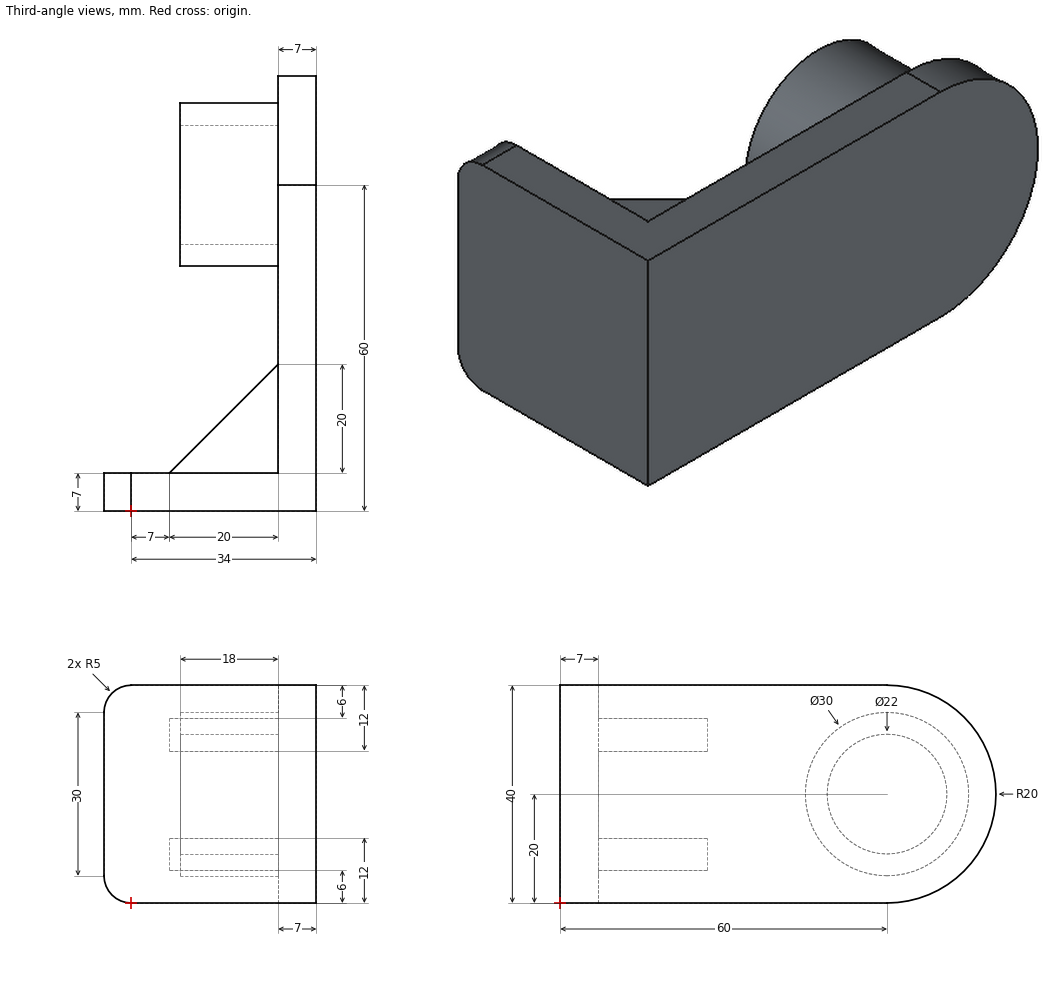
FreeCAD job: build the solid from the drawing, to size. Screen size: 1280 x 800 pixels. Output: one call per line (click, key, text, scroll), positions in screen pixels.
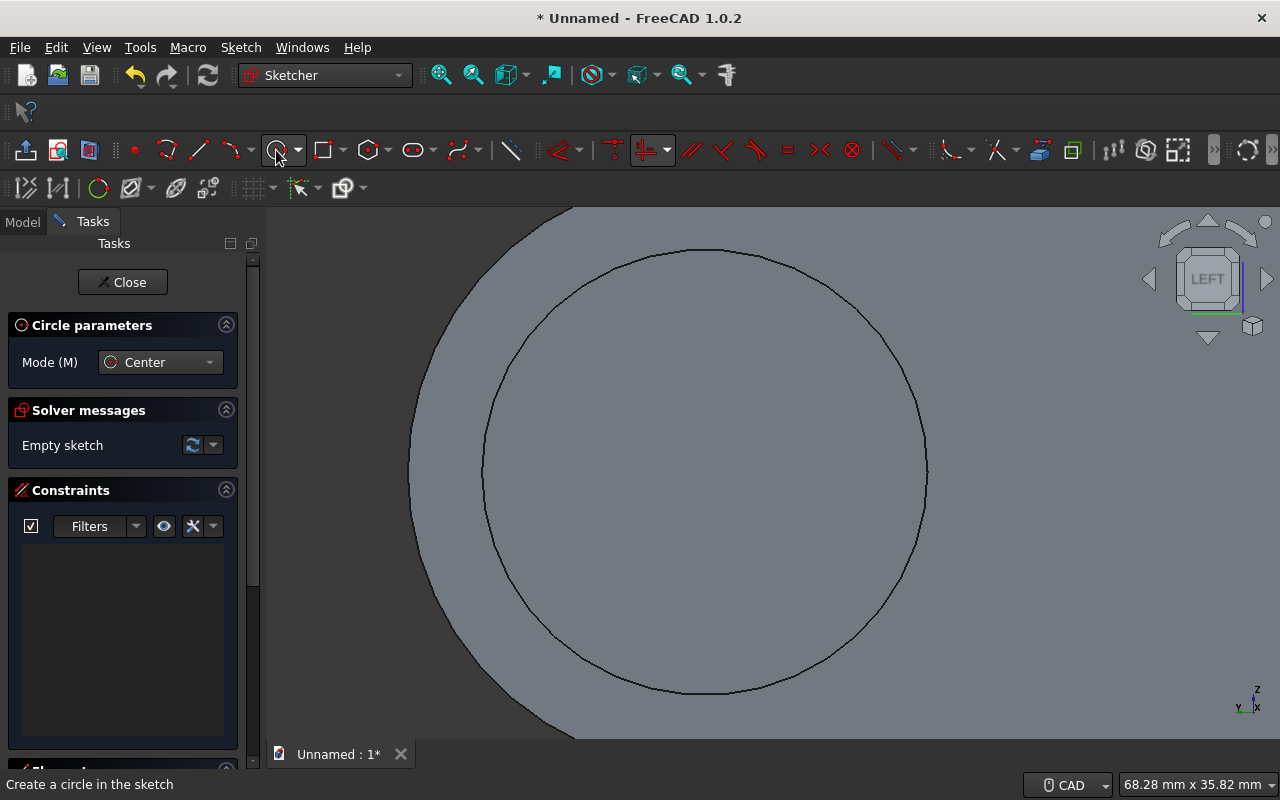
click(705, 472)
click(820, 357)
key(Escape)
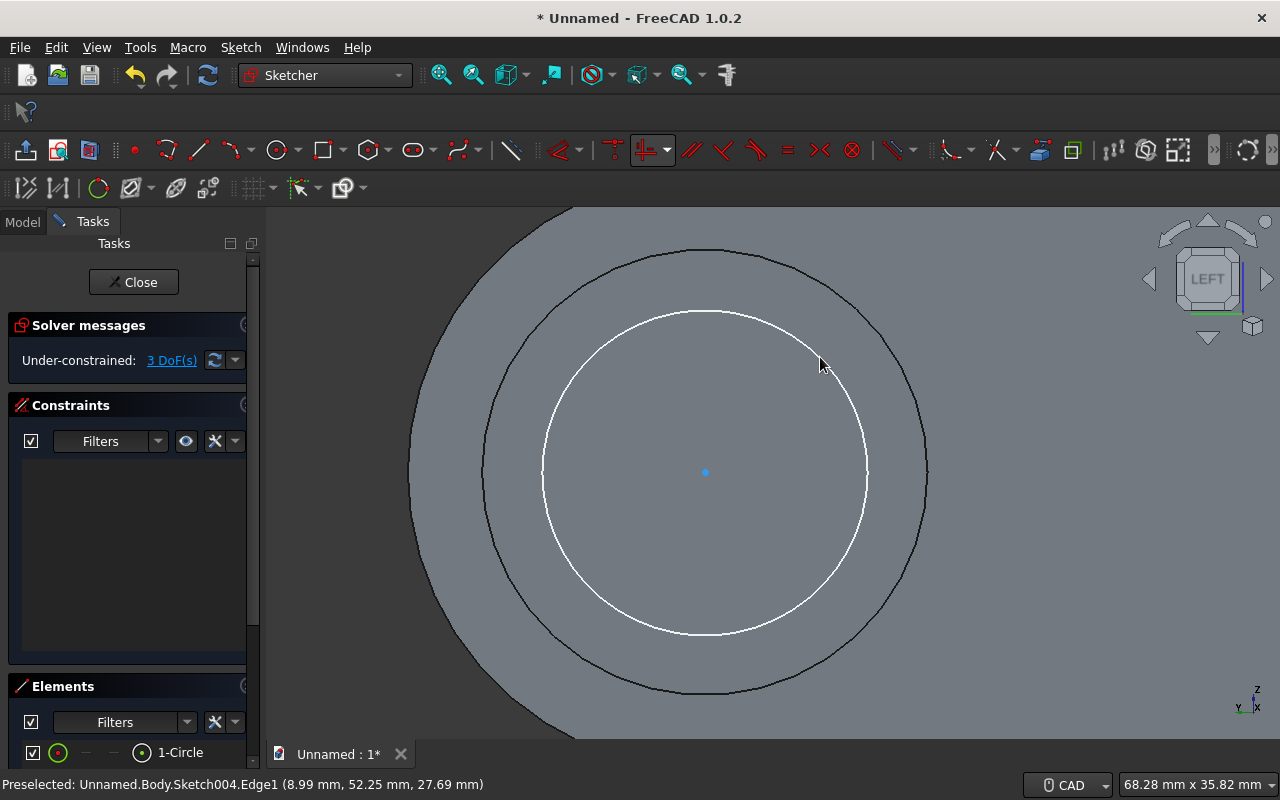
click(558, 150)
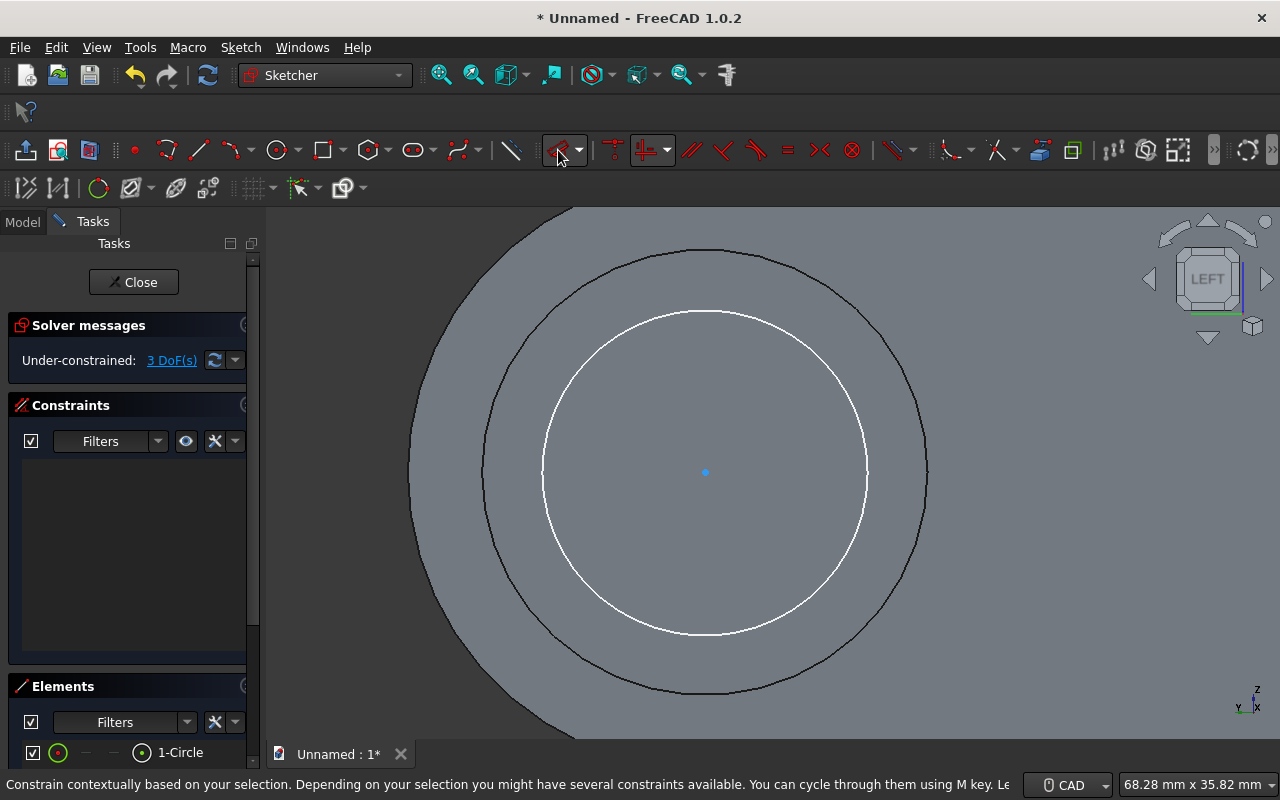
click(820, 358)
click(843, 335)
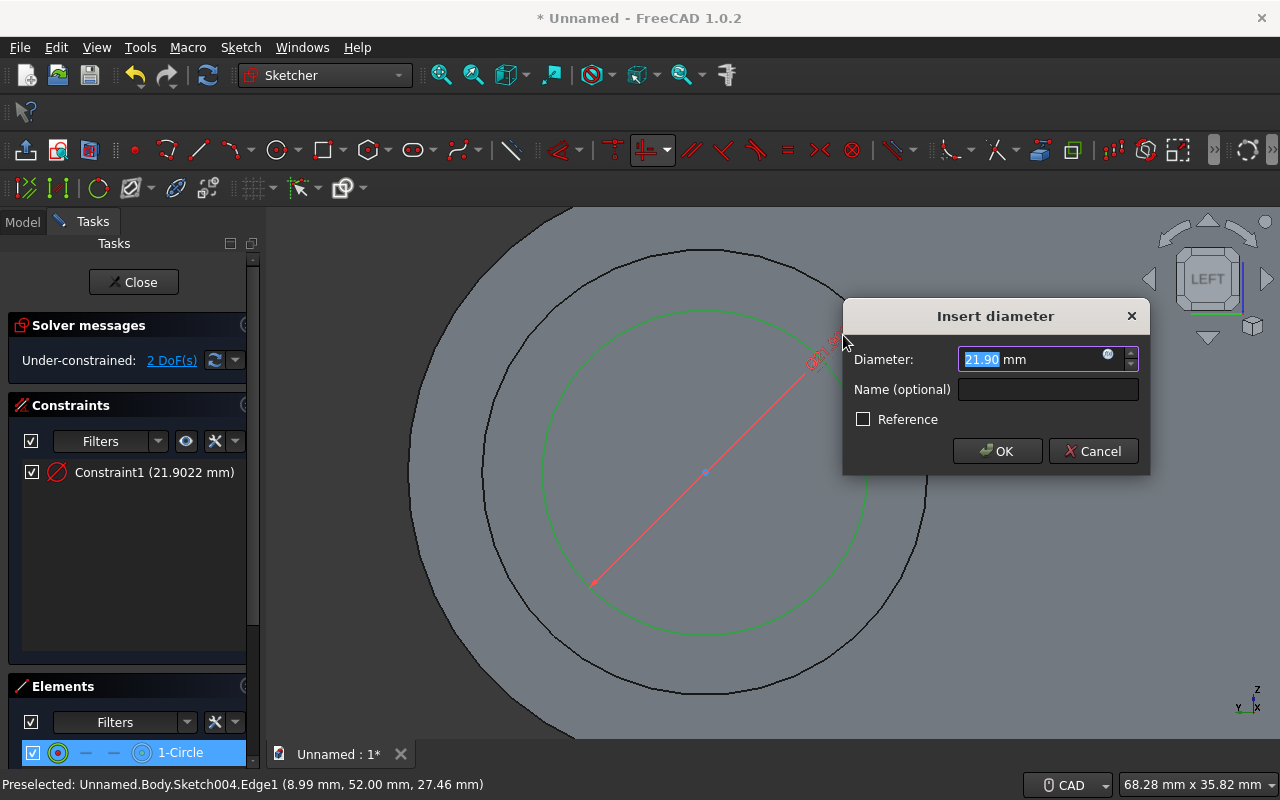
text(22)
key(Return)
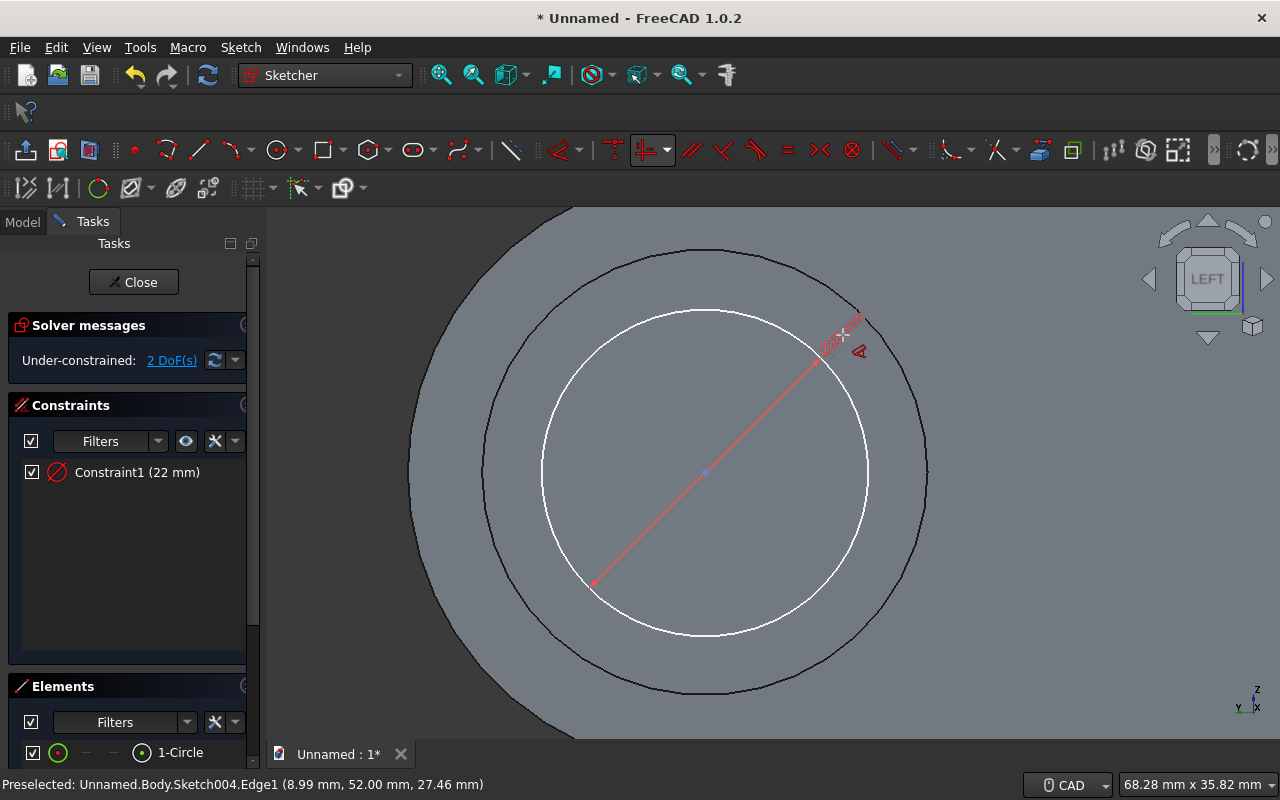
click(705, 473)
click(910, 439)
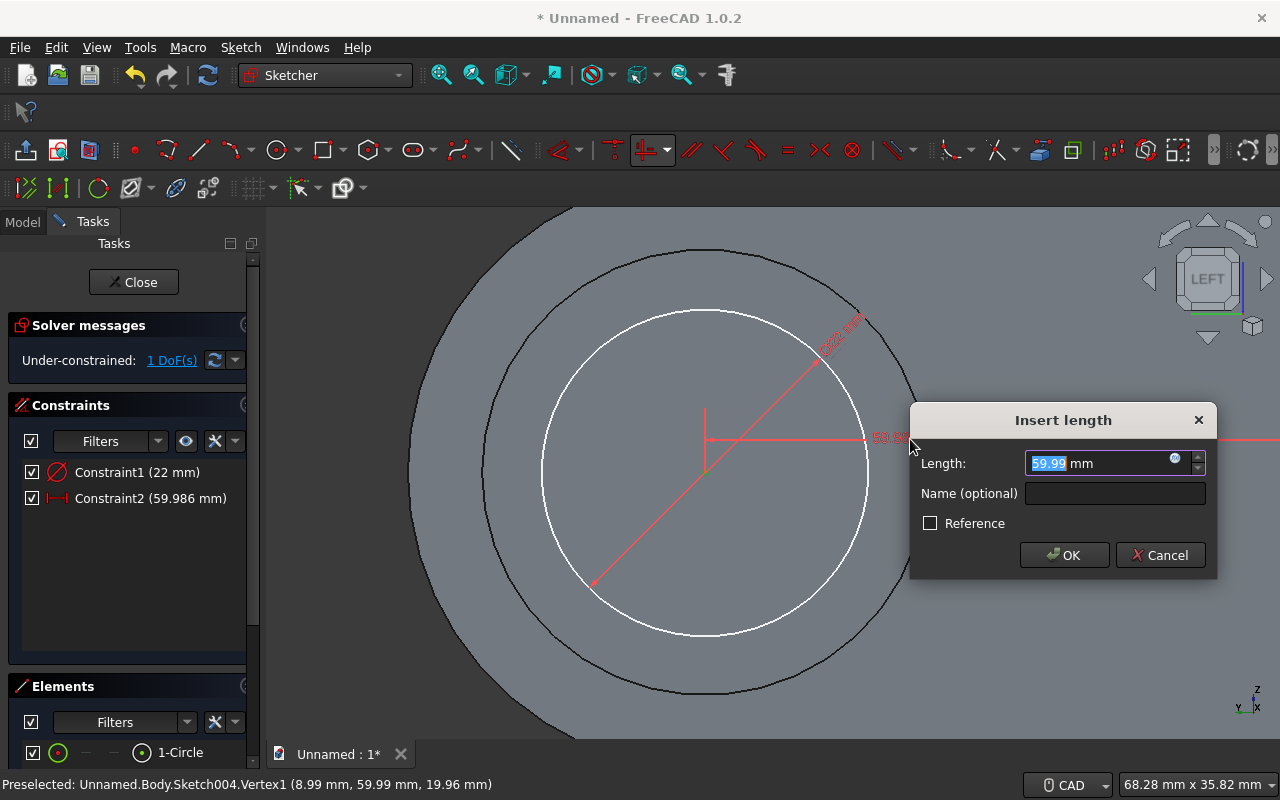
text(60)
key(Return)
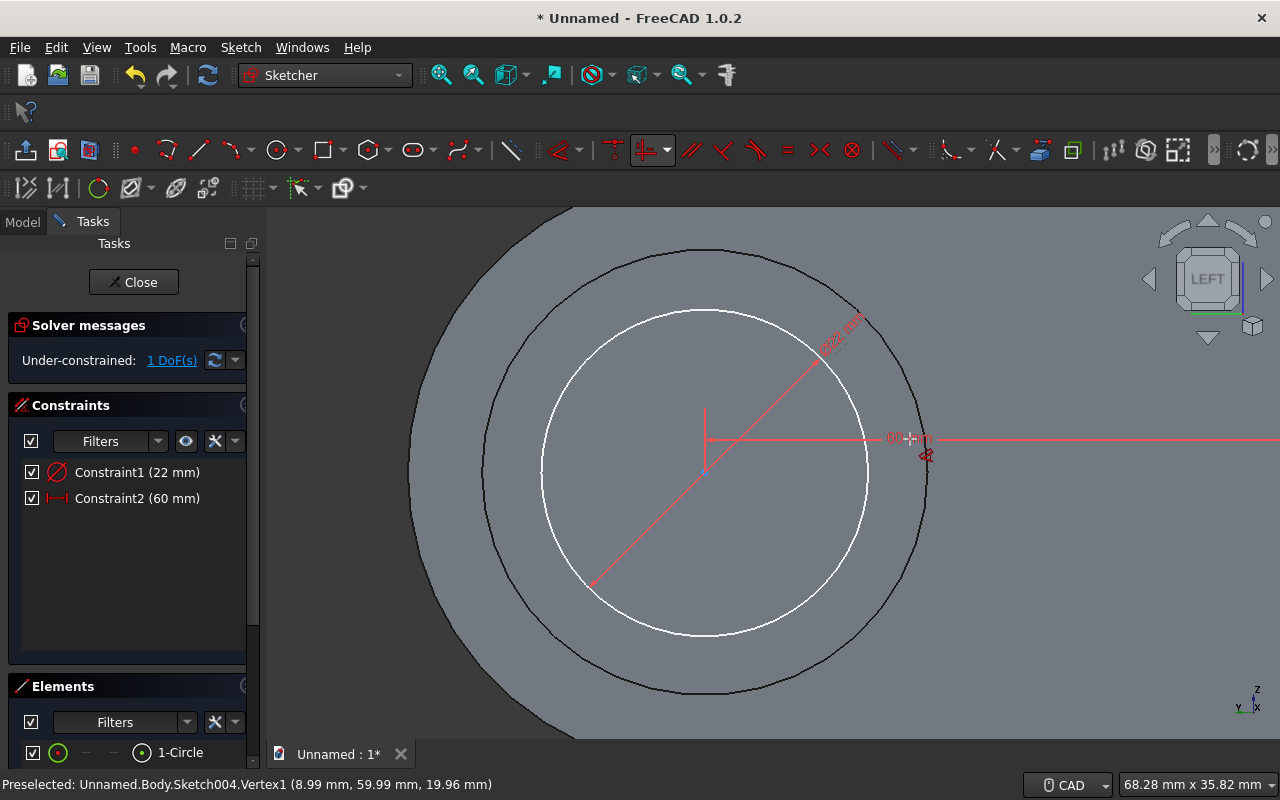
click(705, 473)
click(671, 592)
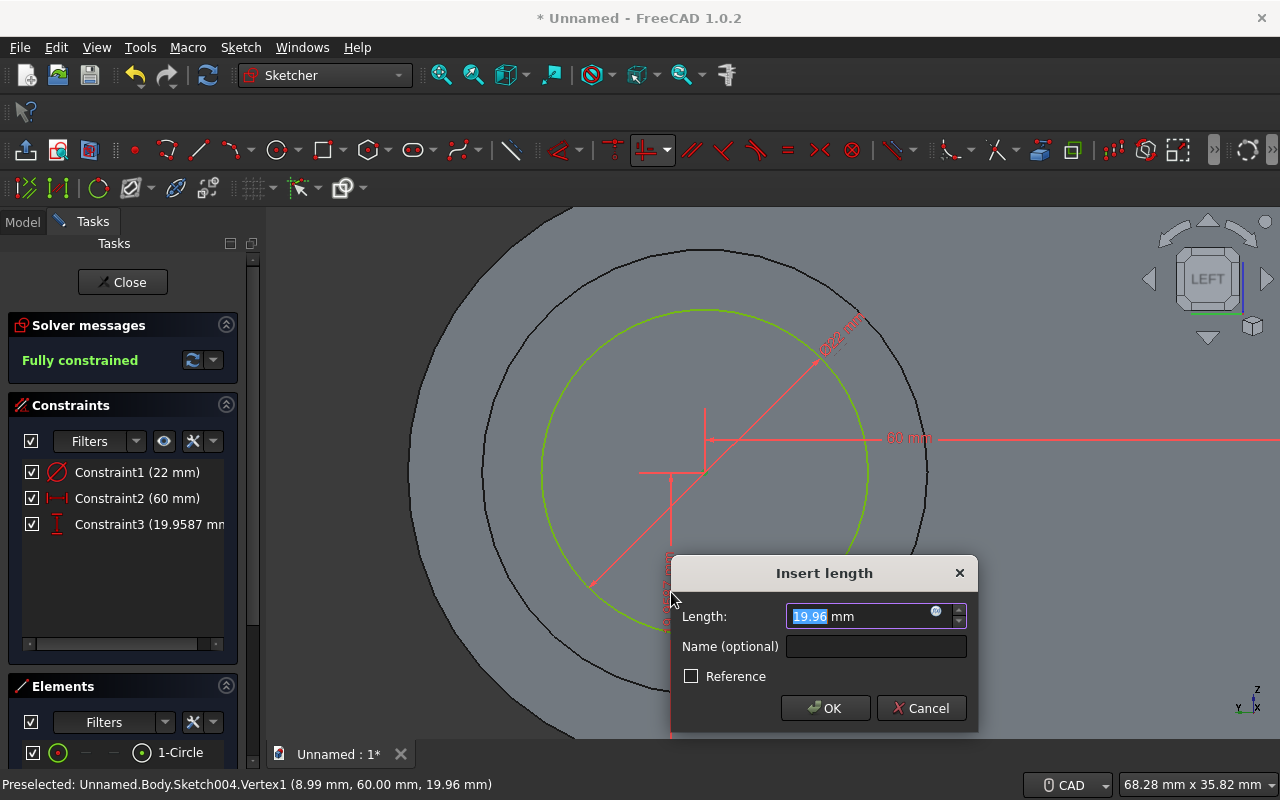
text(20)
key(Return)
key(Escape)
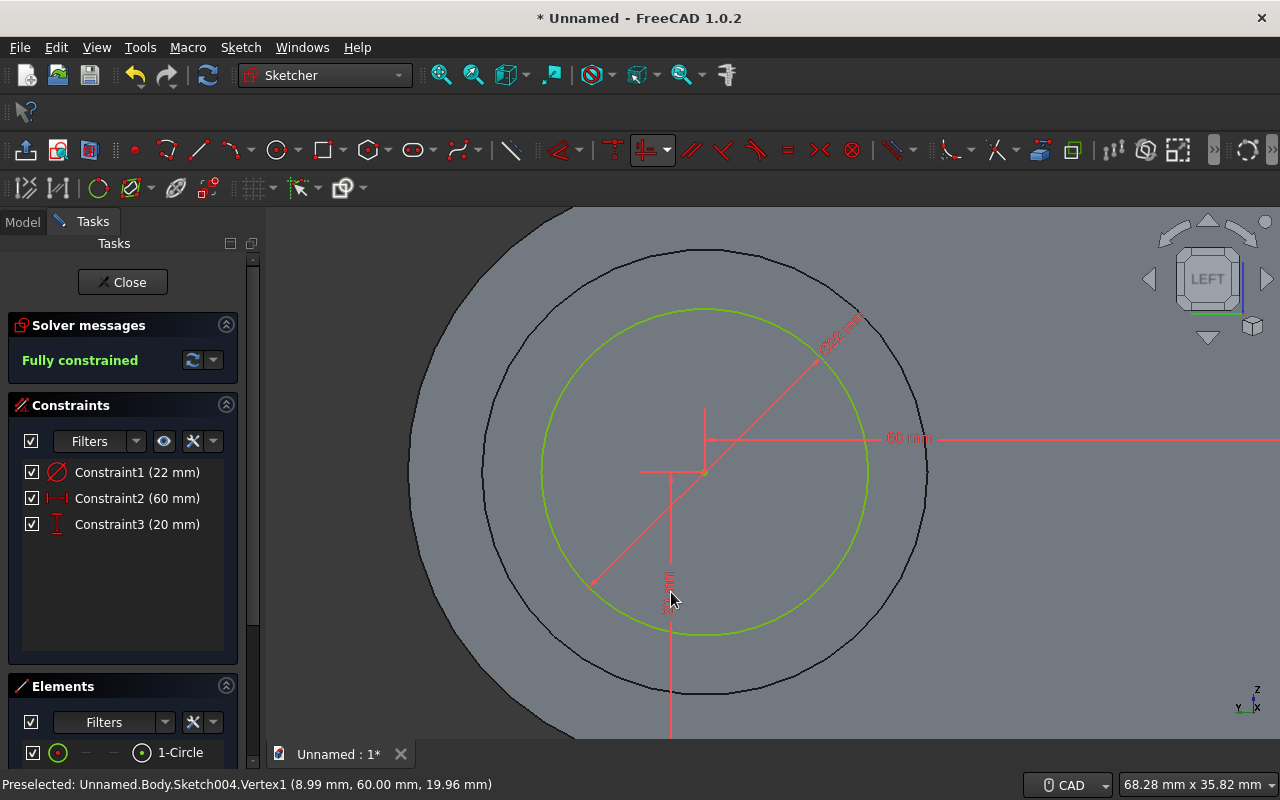
click(123, 282)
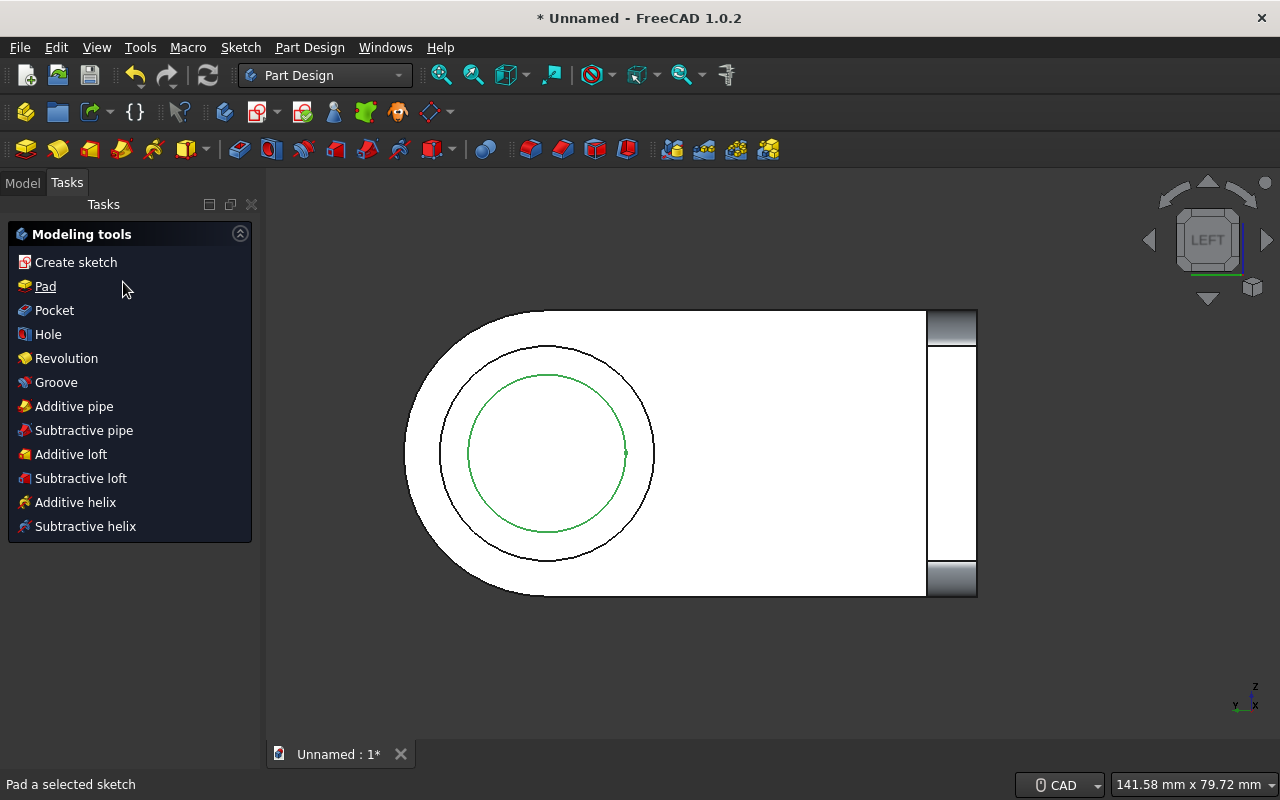
click(240, 150)